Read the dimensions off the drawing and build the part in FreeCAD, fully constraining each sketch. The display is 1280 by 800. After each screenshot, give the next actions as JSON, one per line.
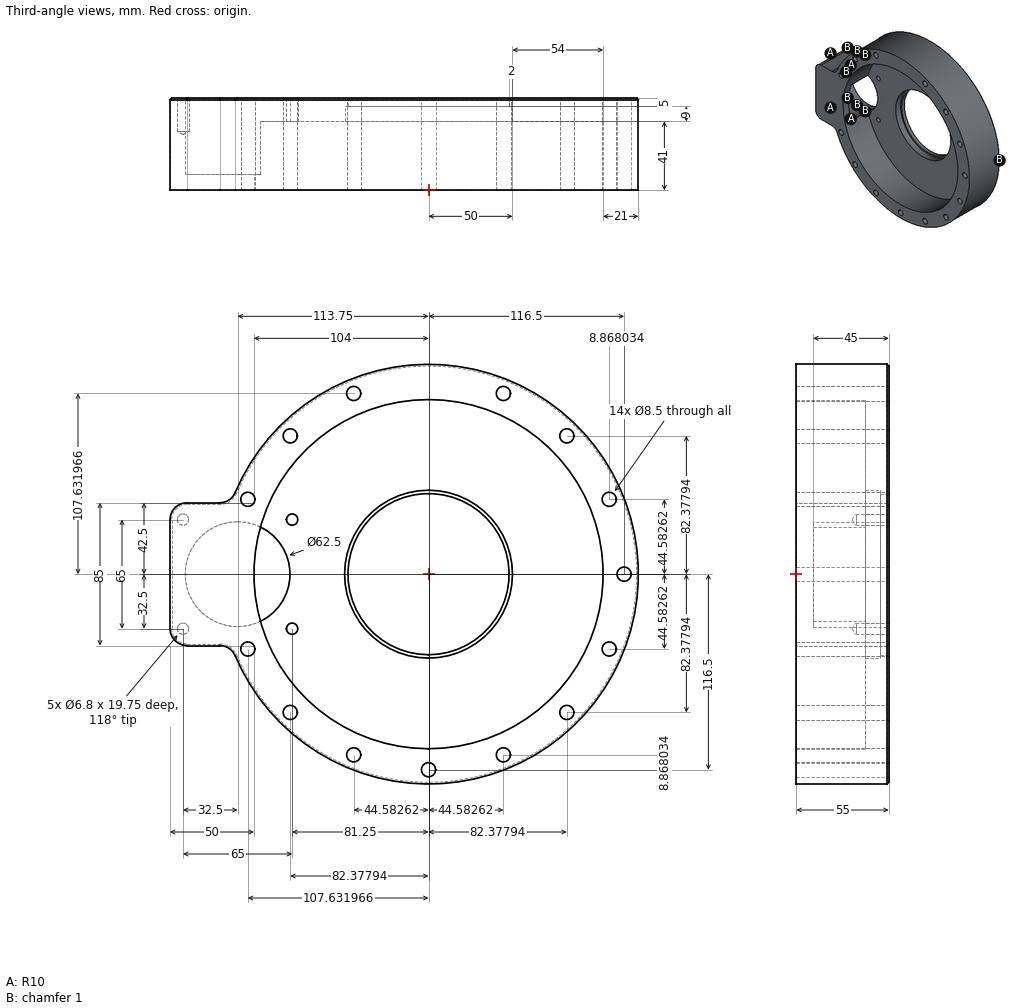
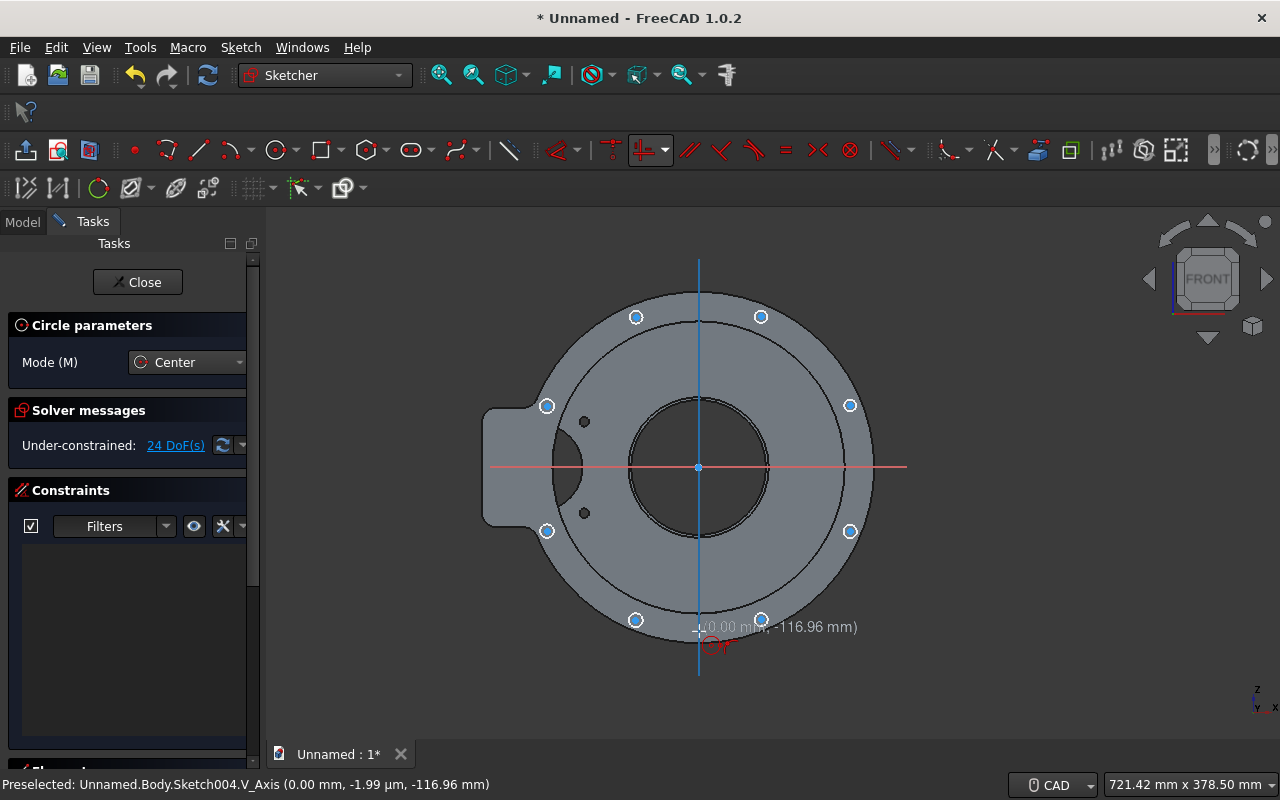
{"action": "left_click", "coordinate": [699, 631]}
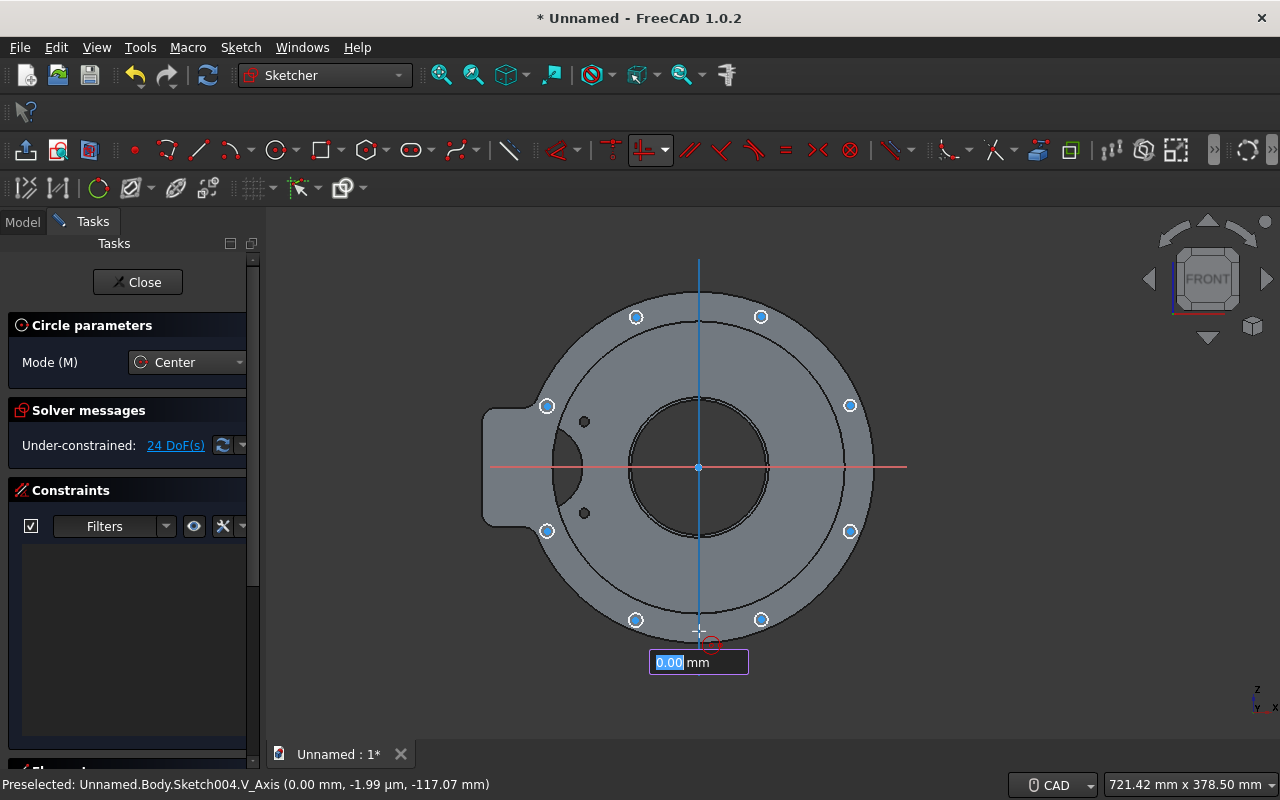
{"action": "scroll", "coordinate": [704, 629], "scroll_direction": "up", "scroll_amount": 6}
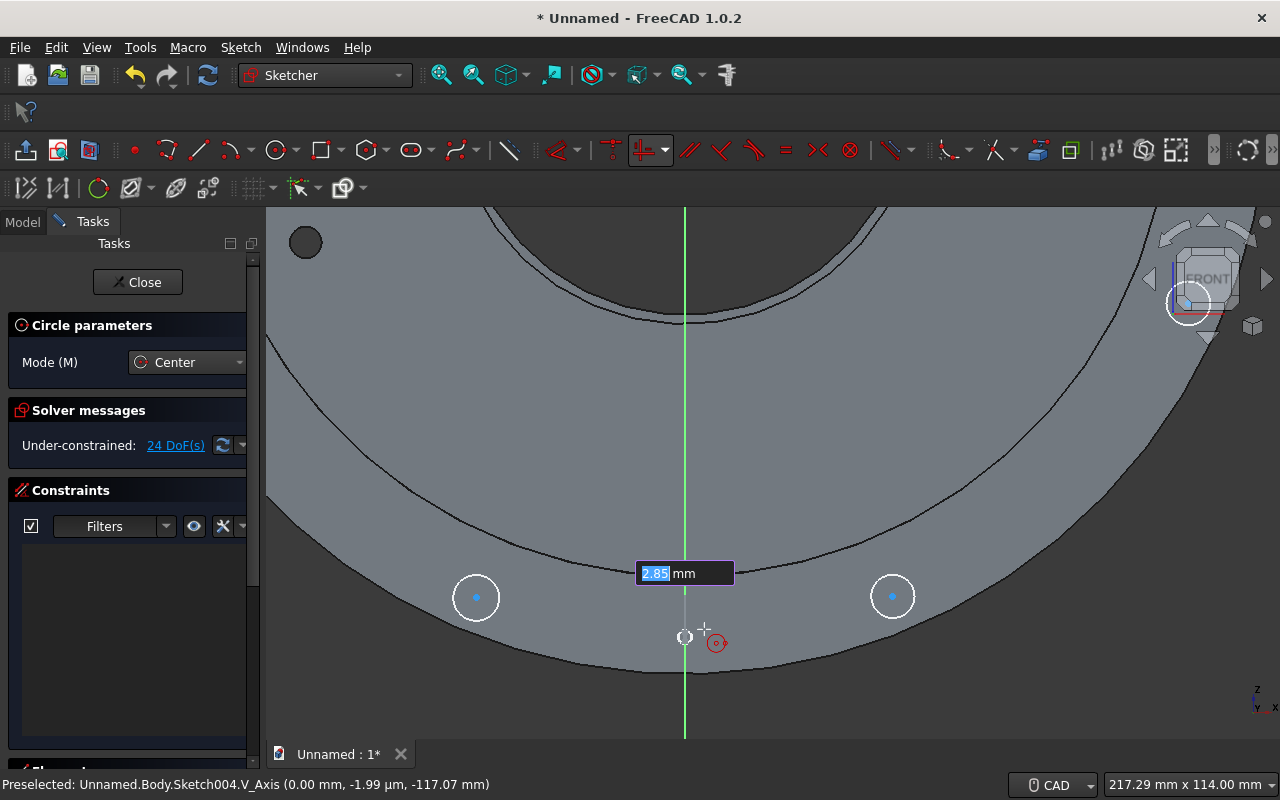
{"action": "left_click", "coordinate": [704, 628]}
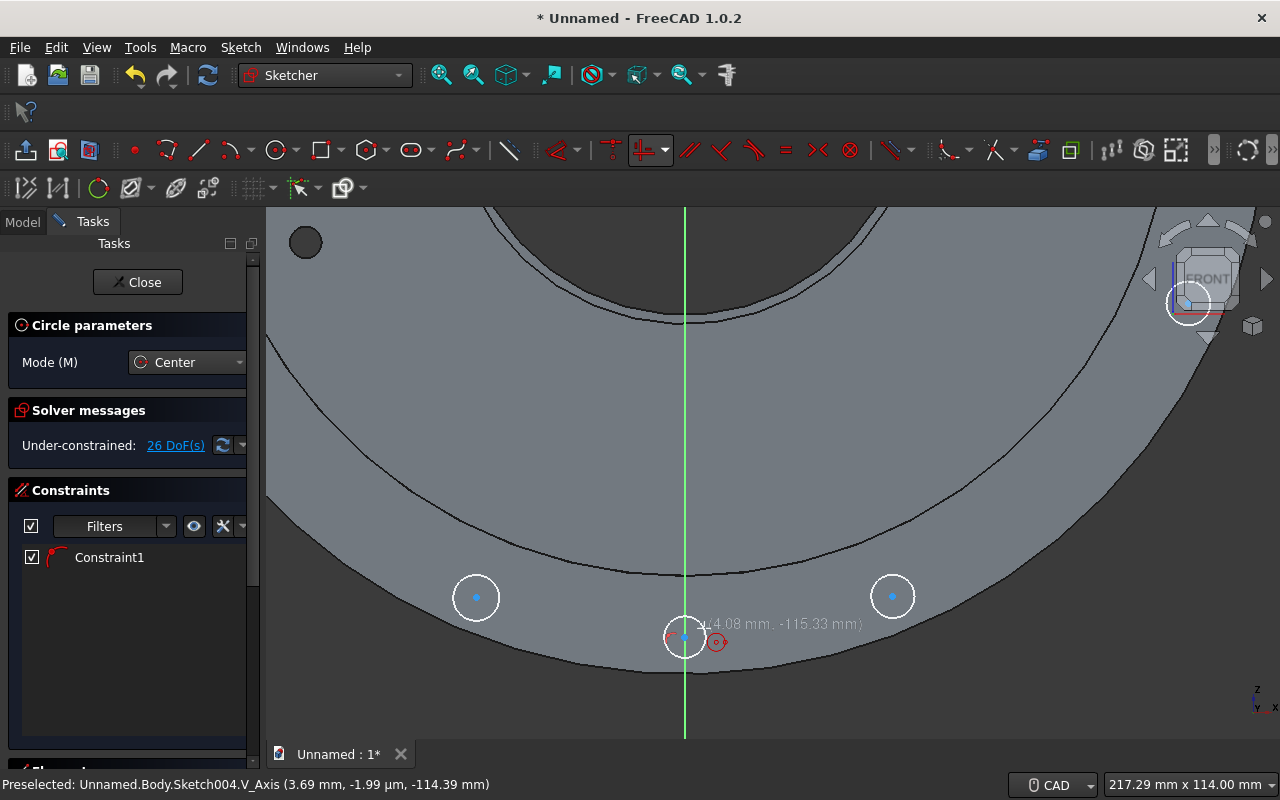
{"action": "left_click", "coordinate": [1069, 475]}
{"action": "left_click", "coordinate": [1083, 461]}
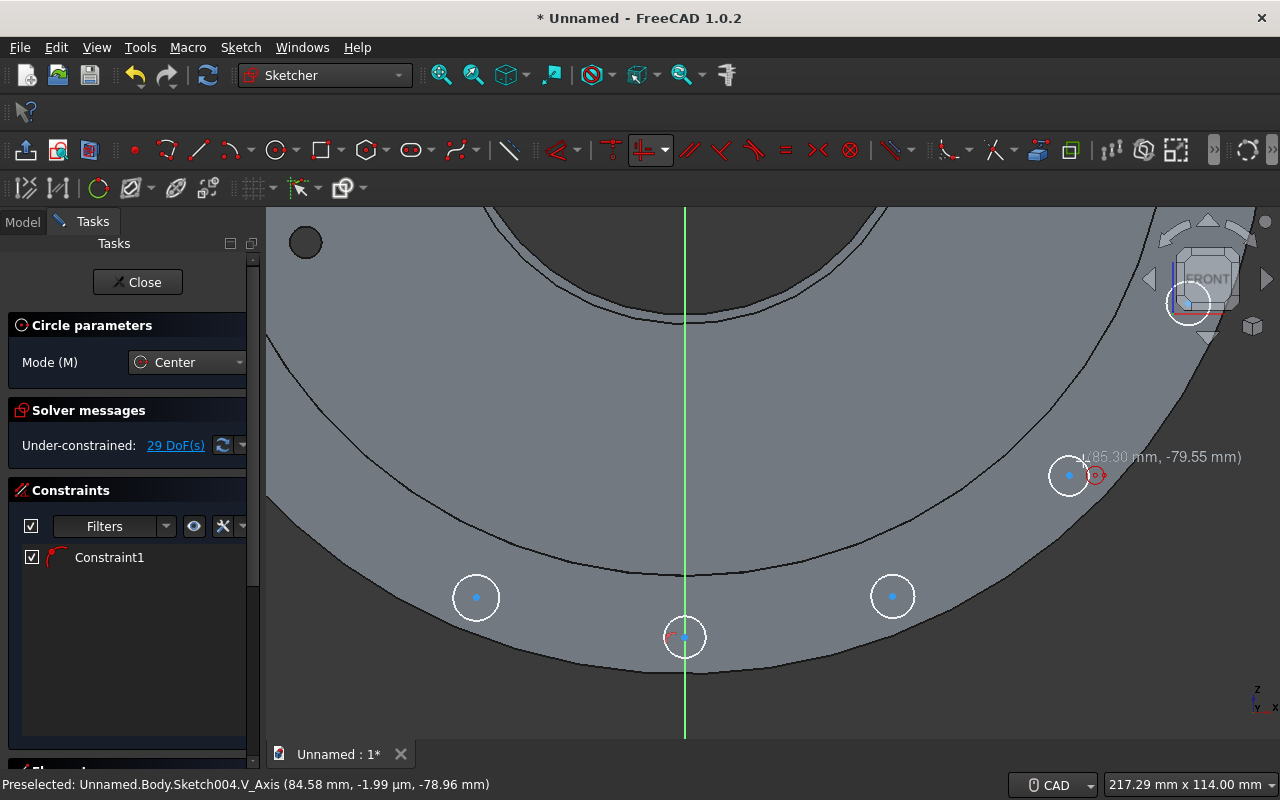
{"action": "left_click", "coordinate": [301, 475]}
{"action": "left_click", "coordinate": [315, 461]}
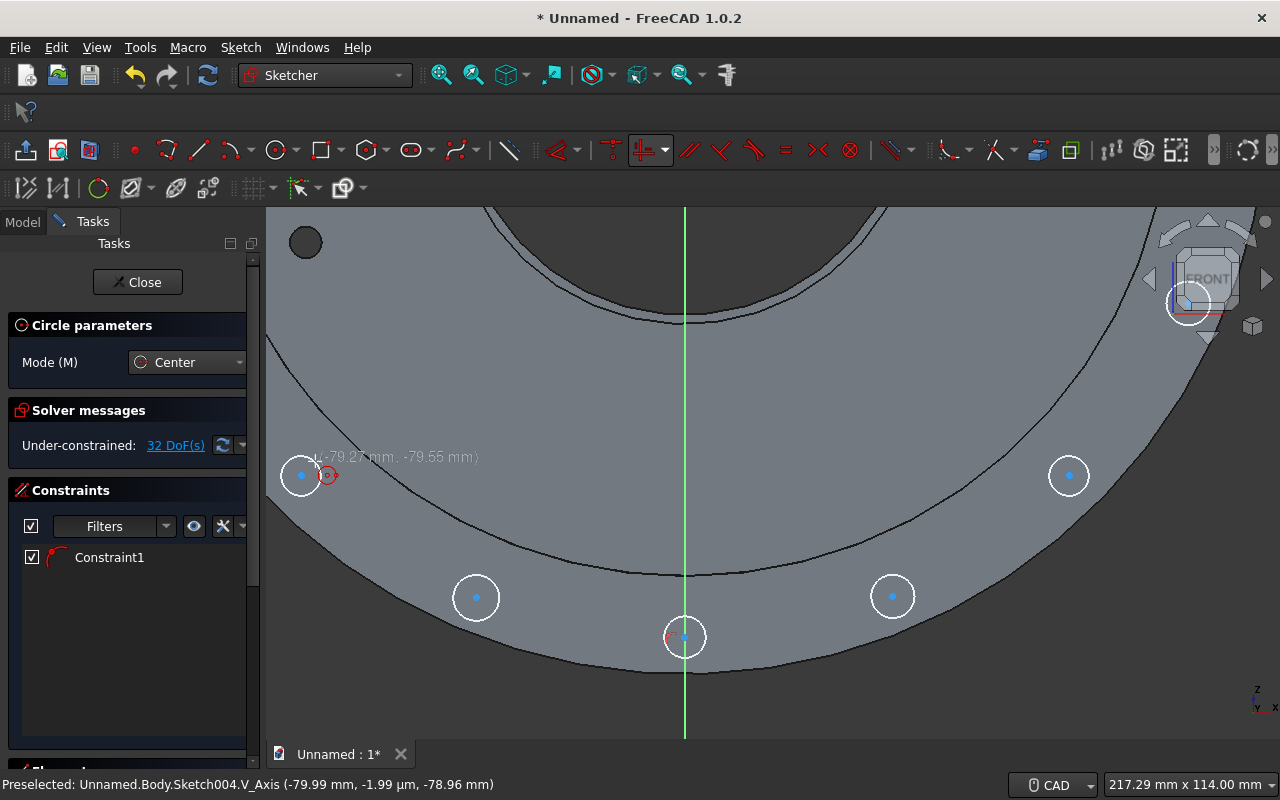
{"action": "scroll", "coordinate": [704, 629], "scroll_direction": "down", "scroll_amount": 6}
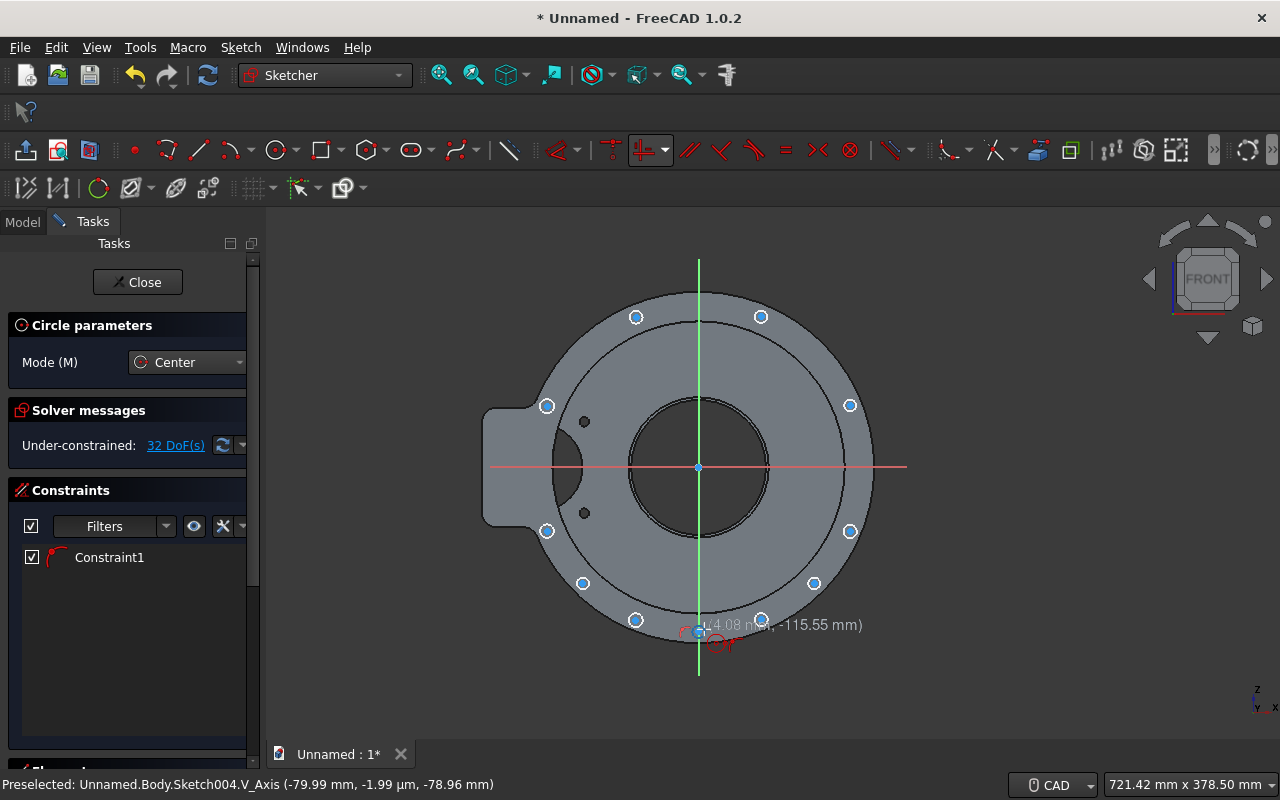
{"action": "scroll", "coordinate": [814, 352], "scroll_direction": "up", "scroll_amount": 7}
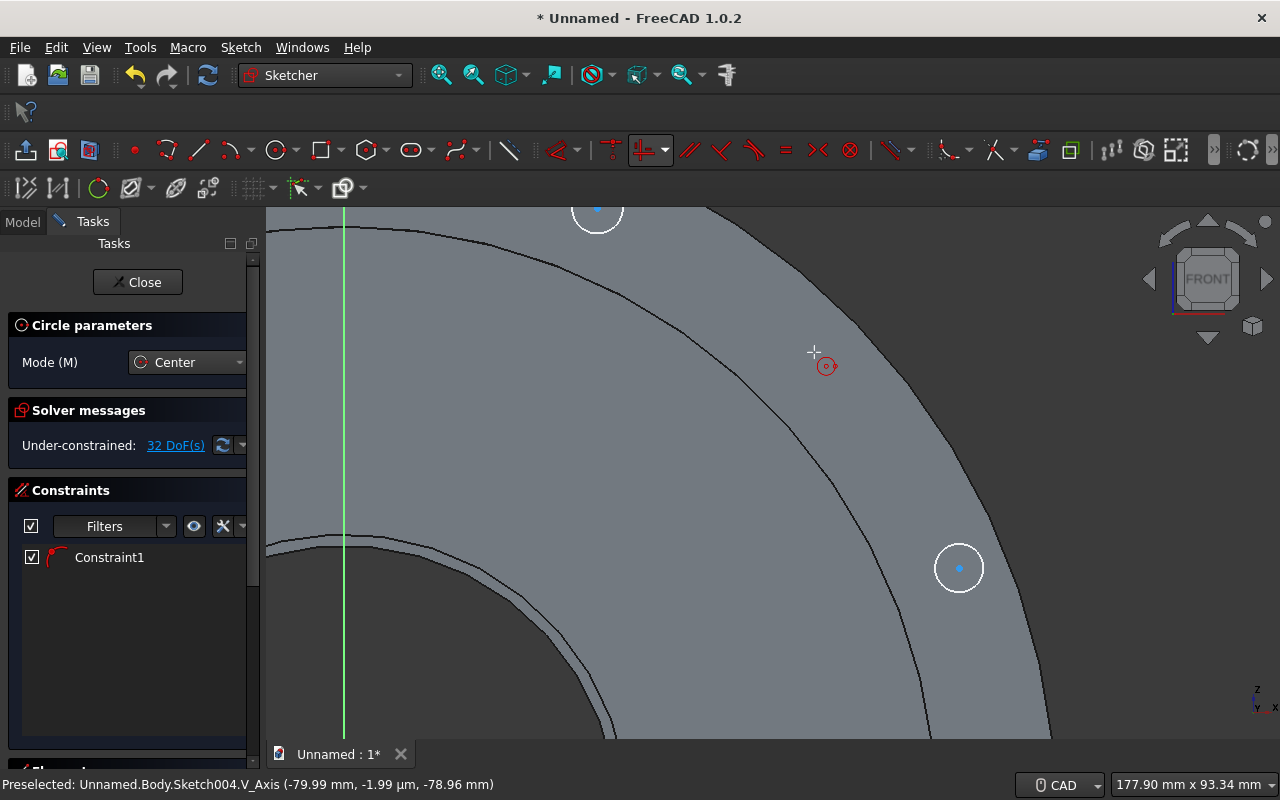
{"action": "scroll", "coordinate": [814, 351], "scroll_direction": "down", "scroll_amount": 7}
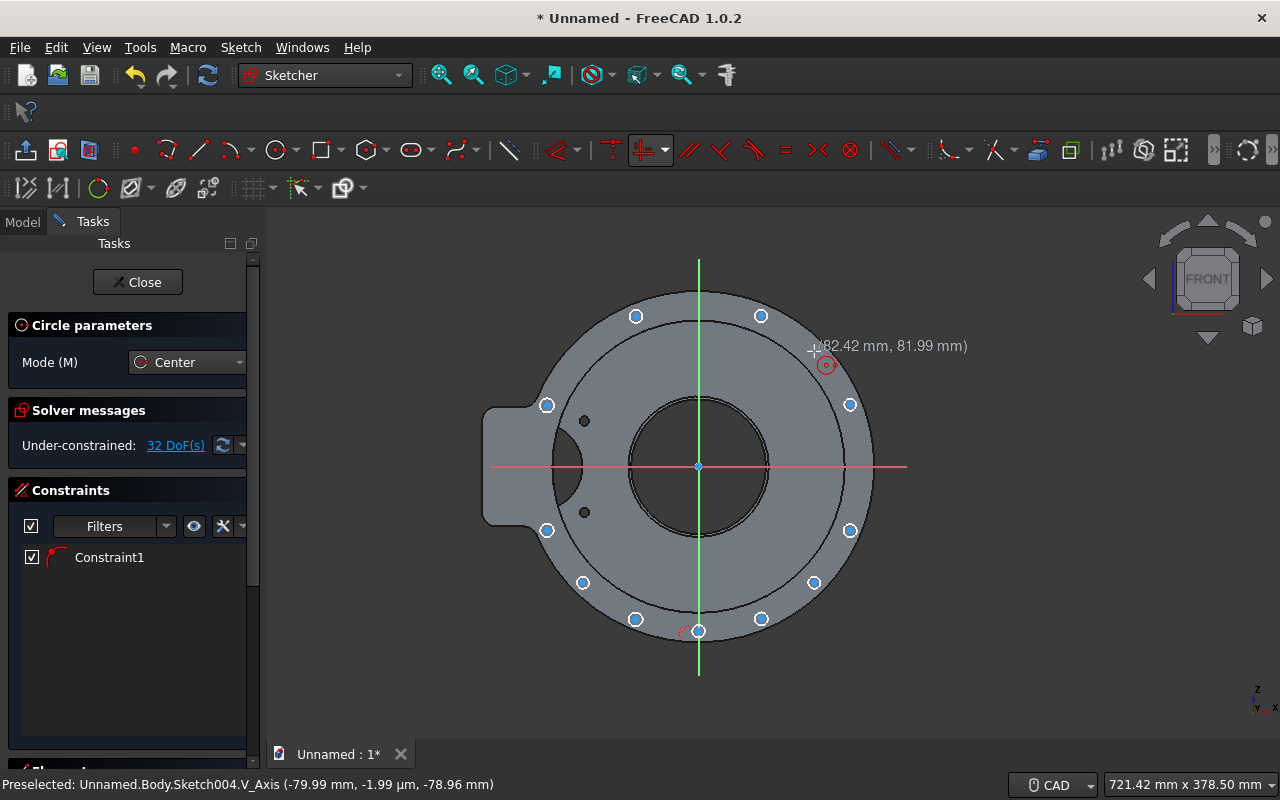
{"action": "left_click", "coordinate": [814, 351]}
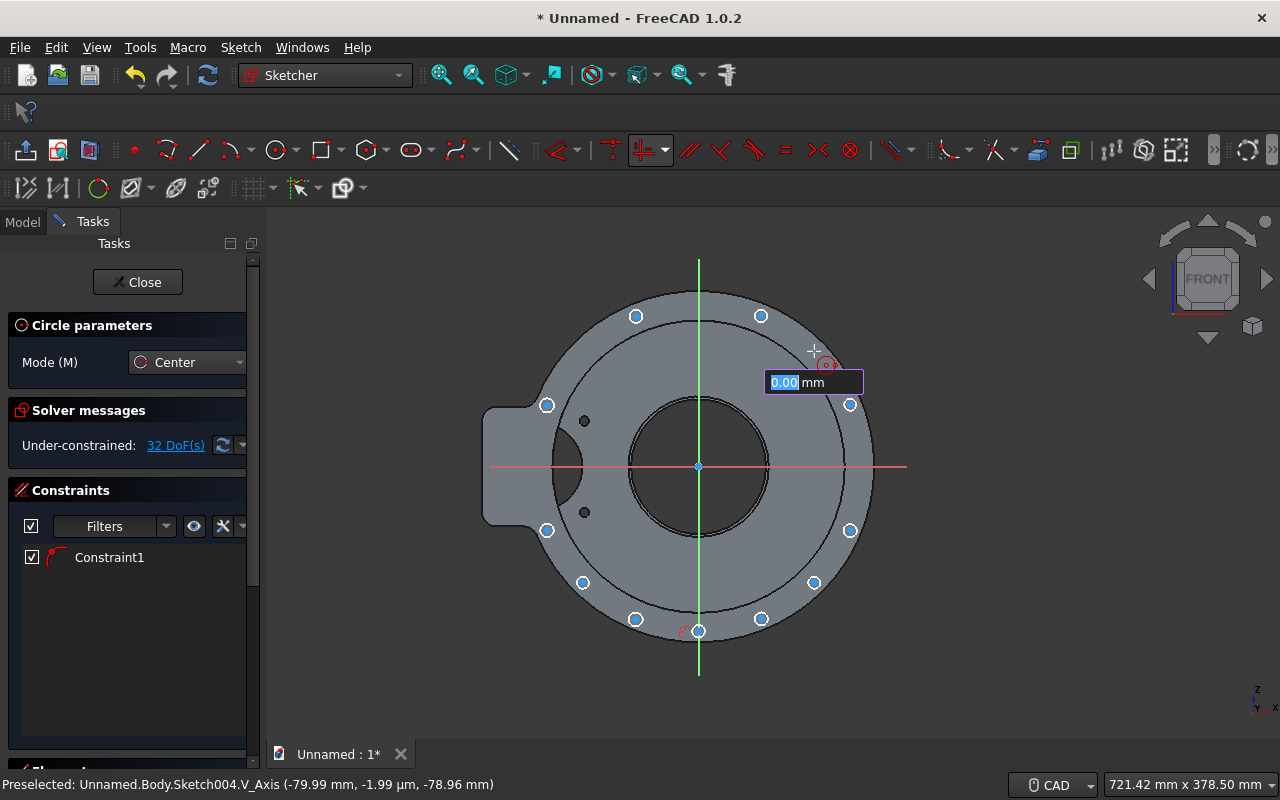
{"action": "scroll", "coordinate": [819, 347], "scroll_direction": "up", "scroll_amount": 5}